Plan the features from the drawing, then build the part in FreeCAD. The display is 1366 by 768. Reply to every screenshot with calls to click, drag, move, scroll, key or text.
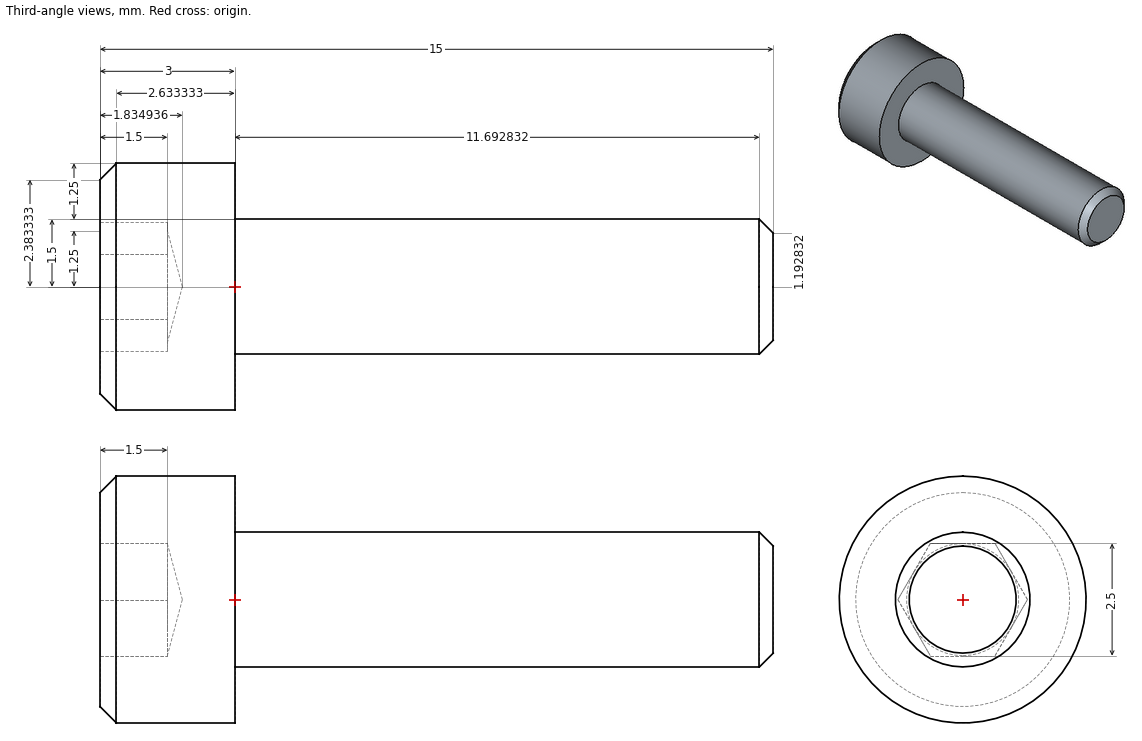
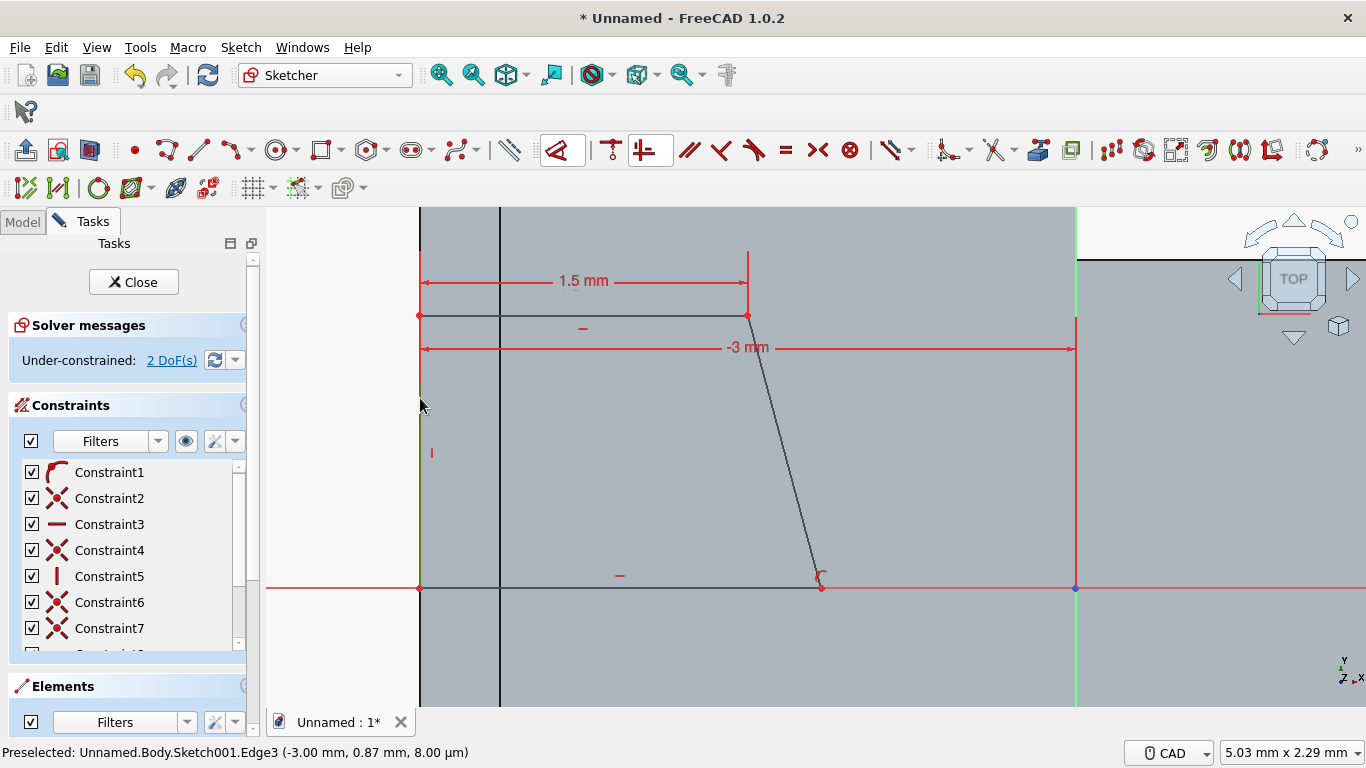
click(580, 150)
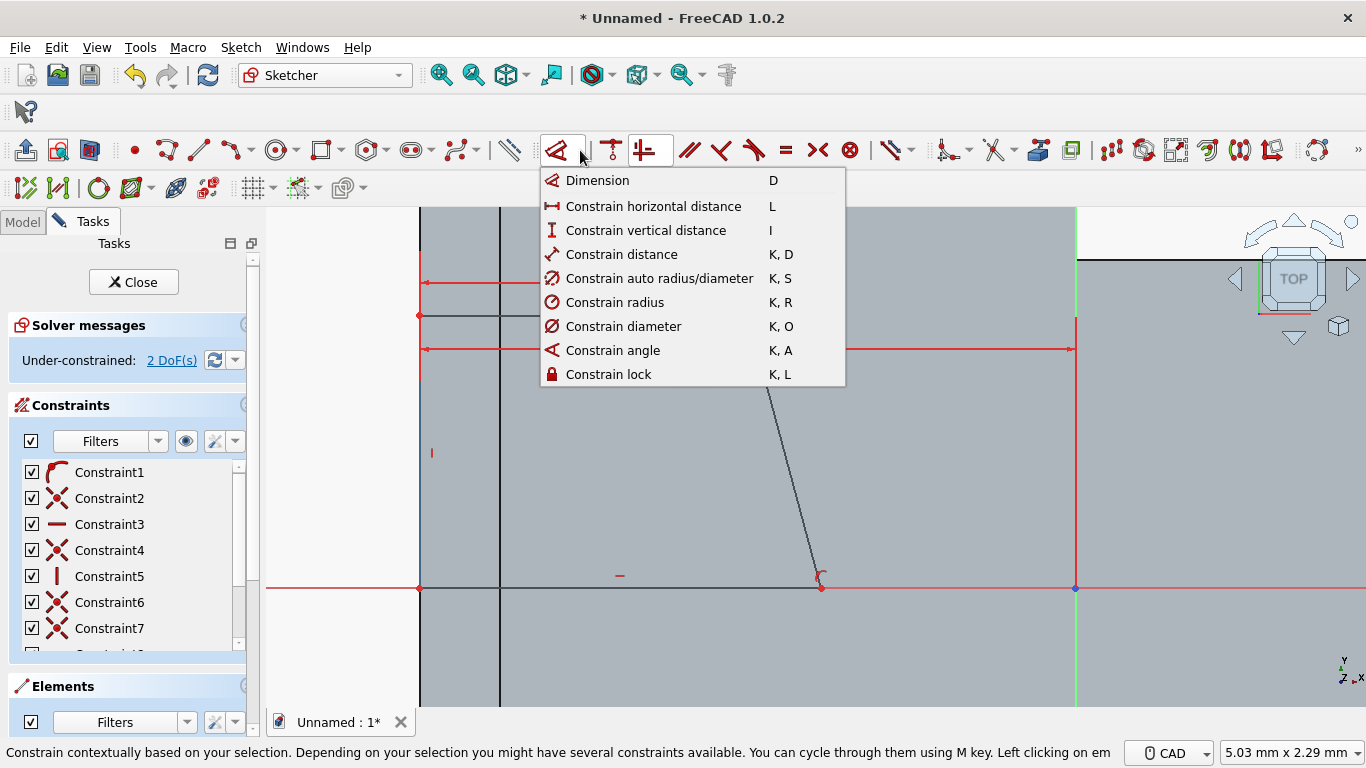
click(693, 230)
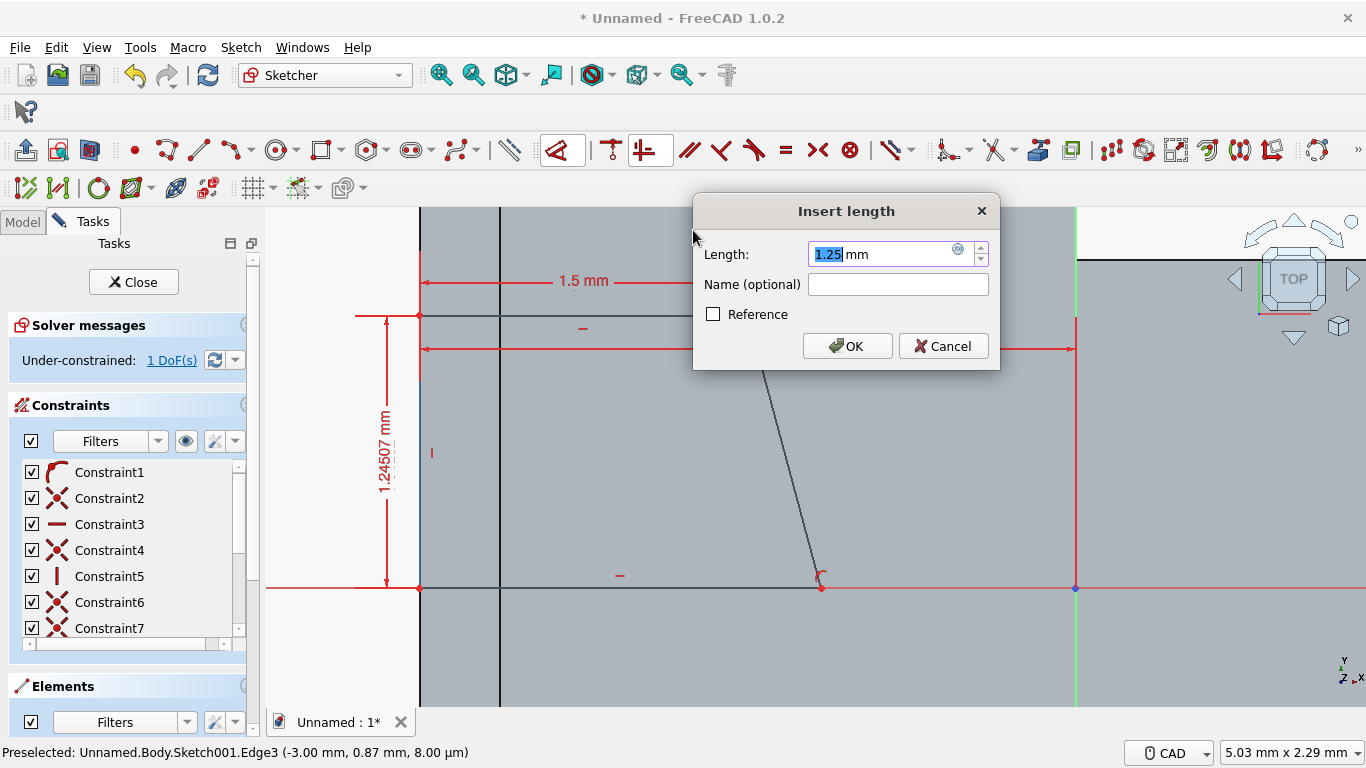
text(1.25)
key(Return)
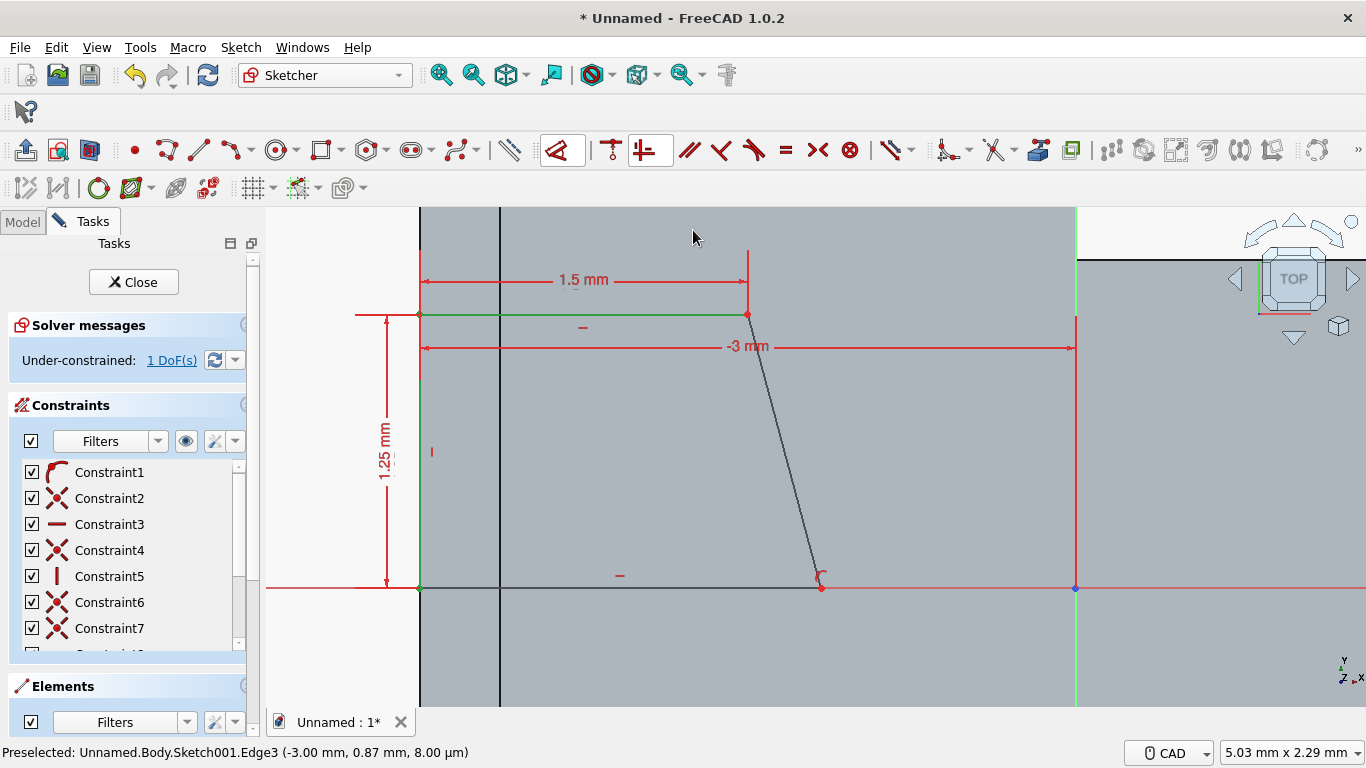
click(540, 588)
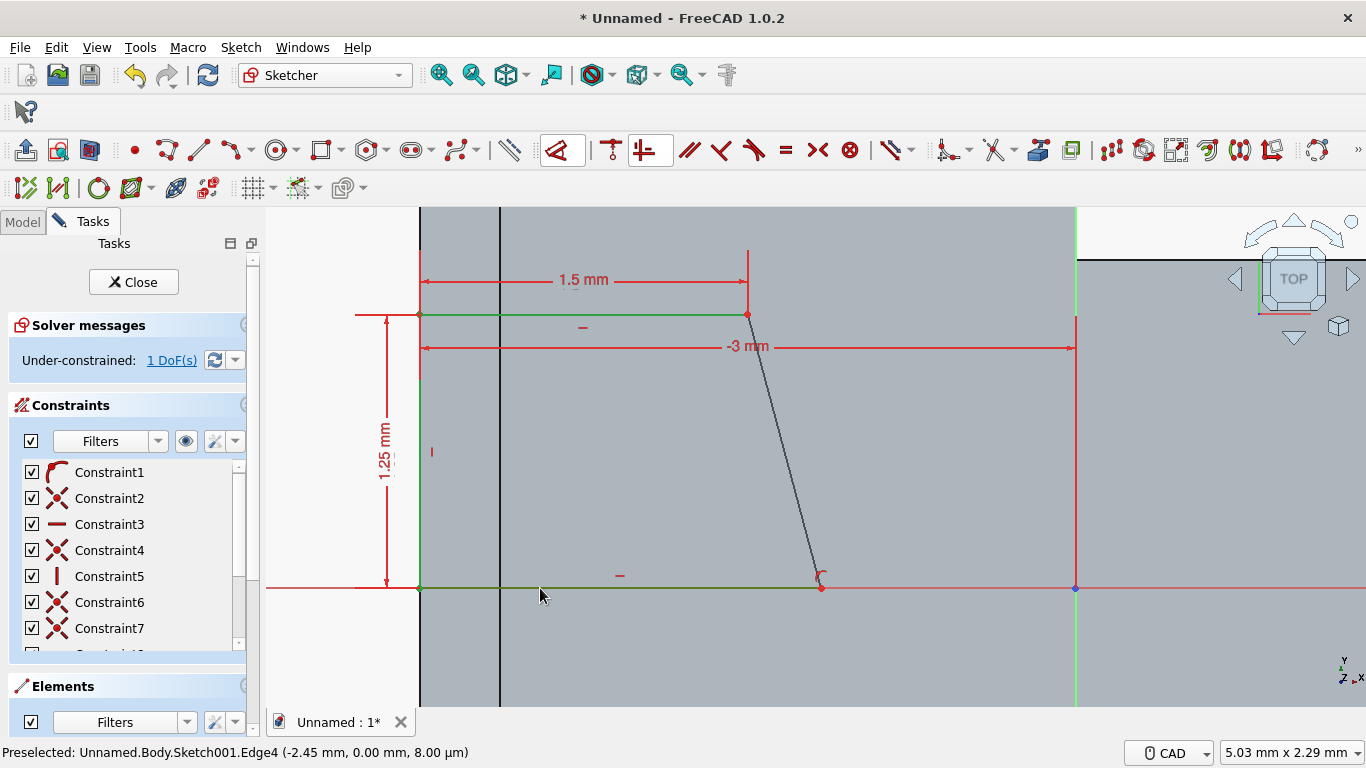
click(580, 150)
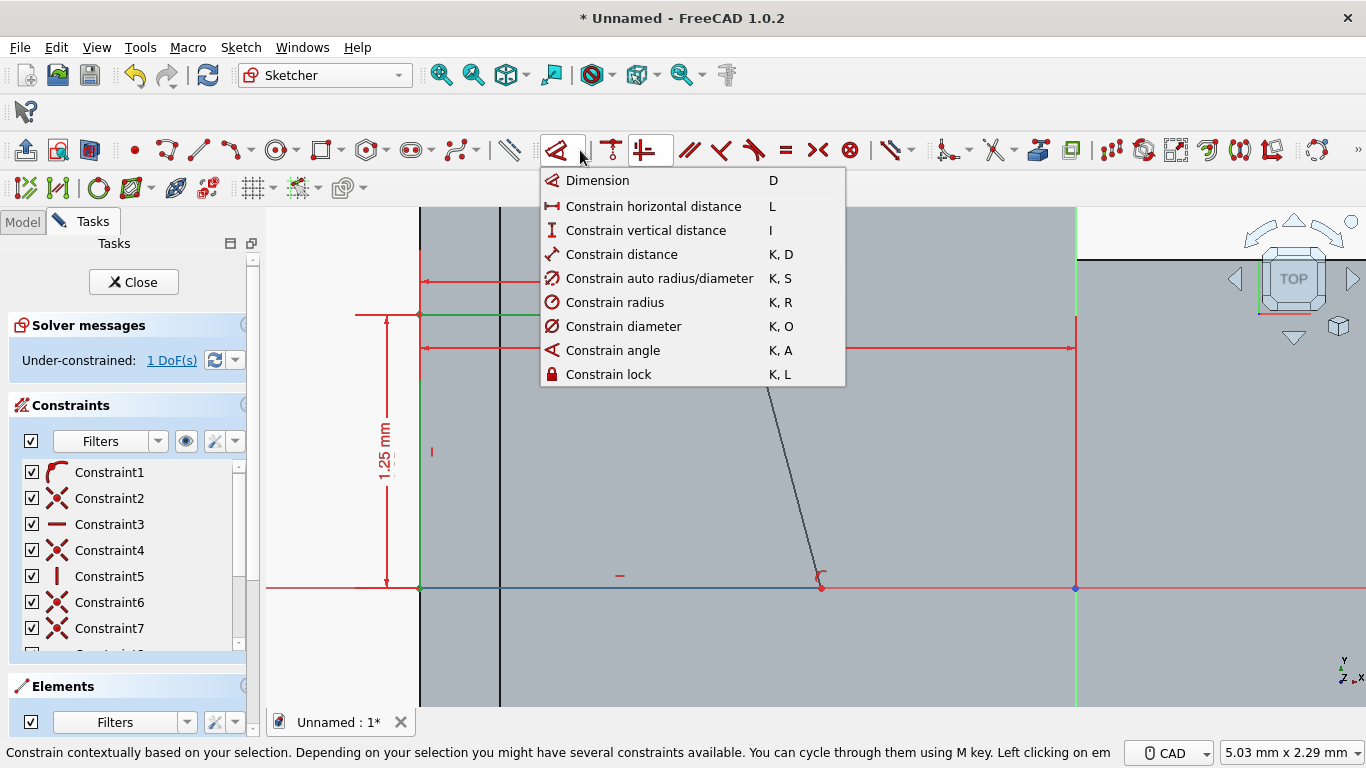
click(693, 206)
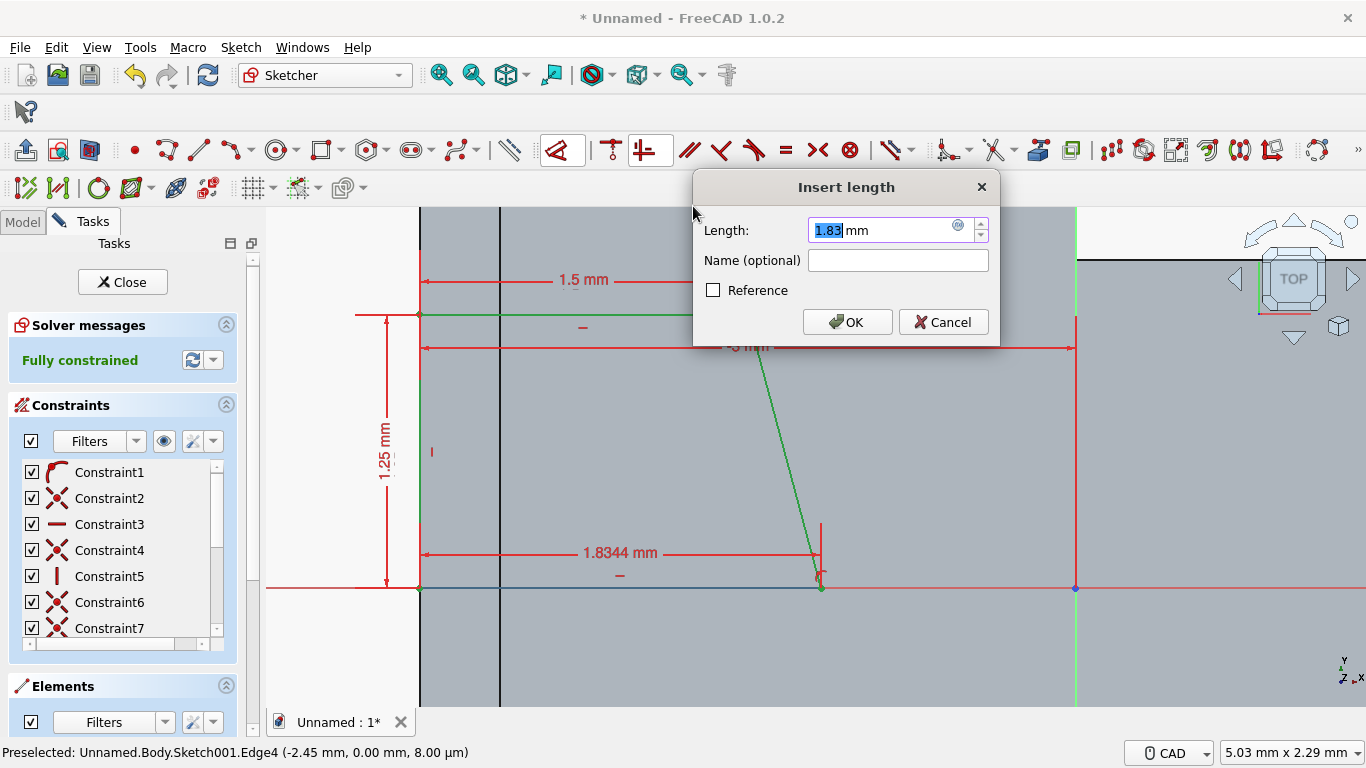
text(1.834936)
key(Return)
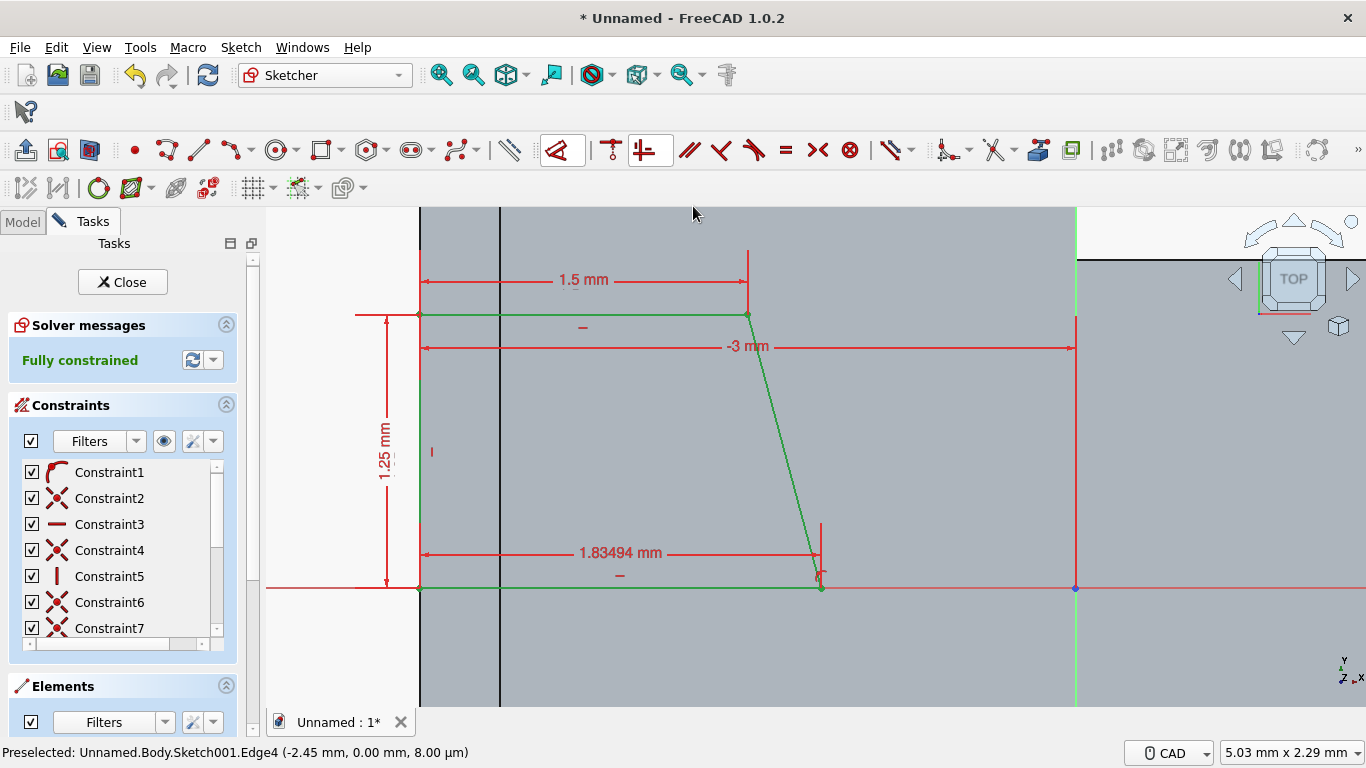
click(123, 282)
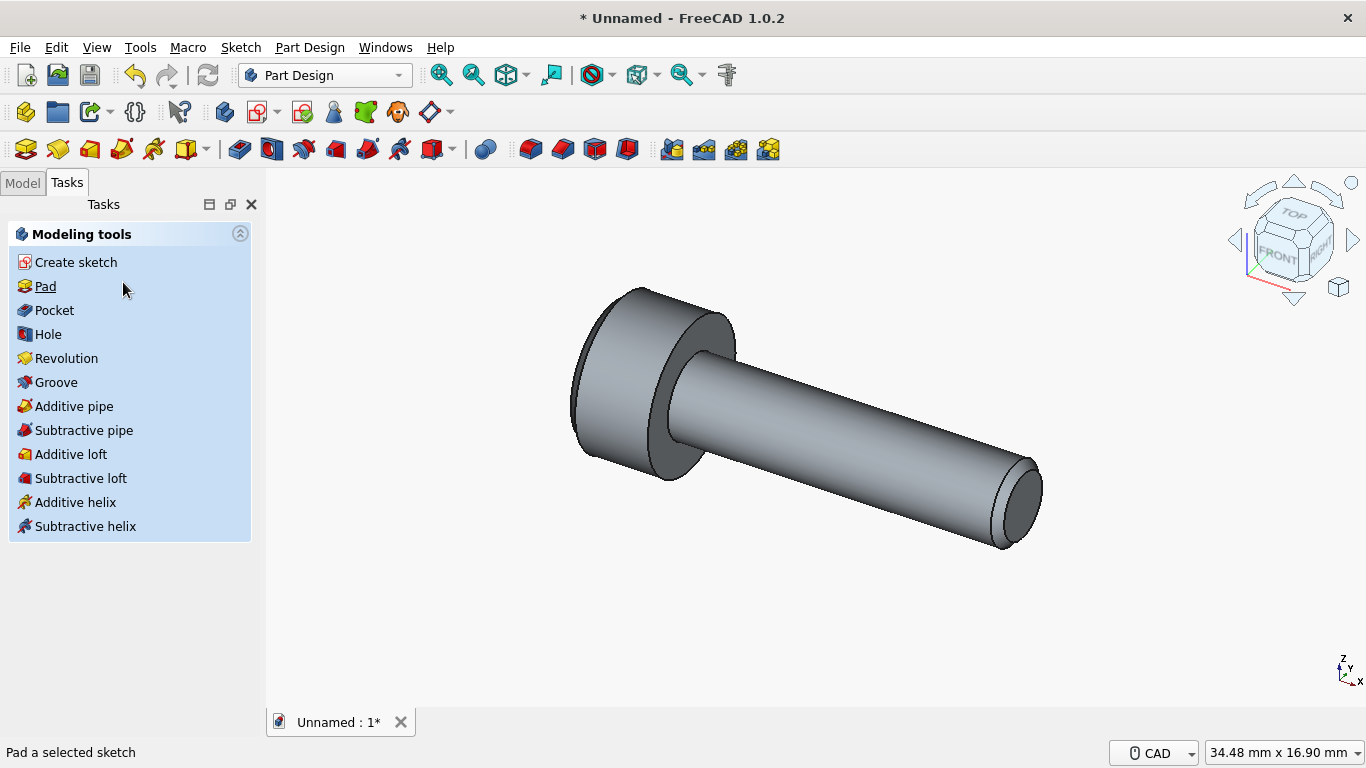
click(304, 150)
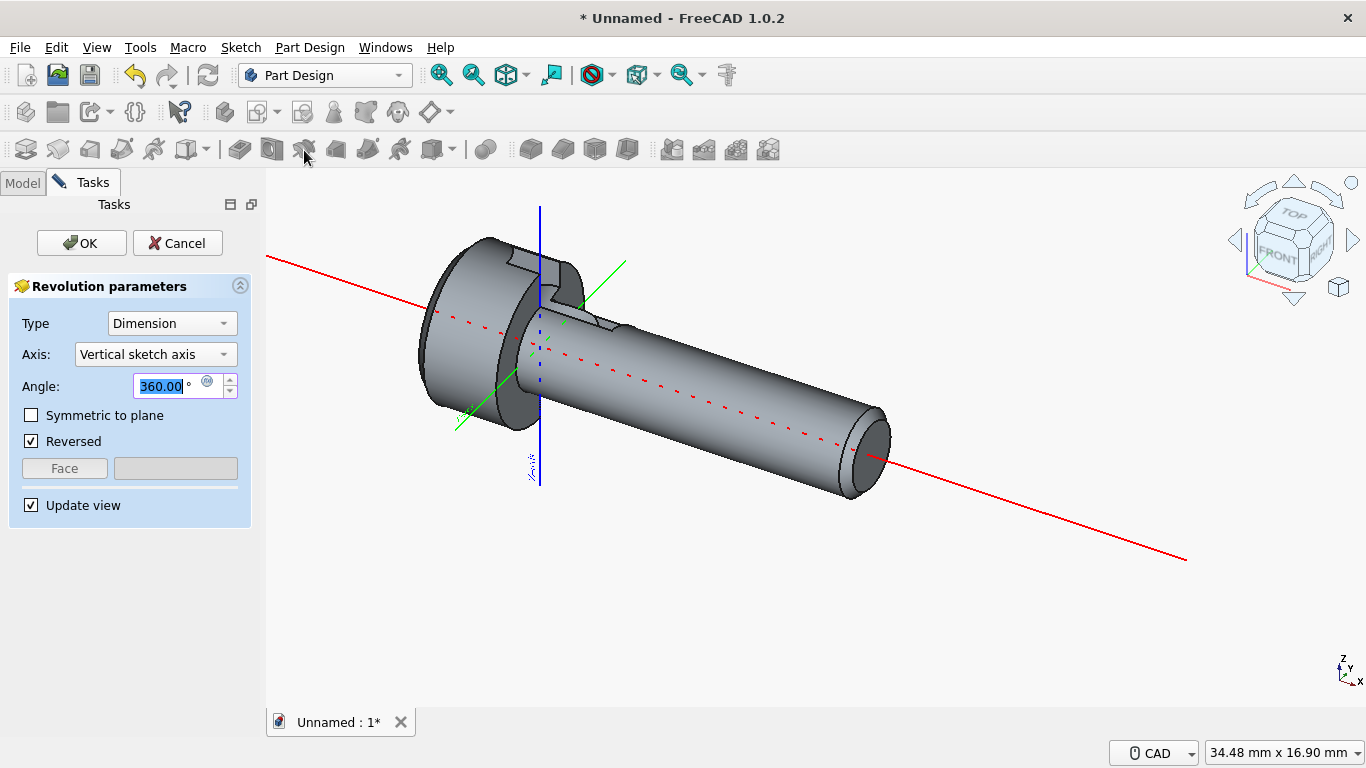
click(156, 354)